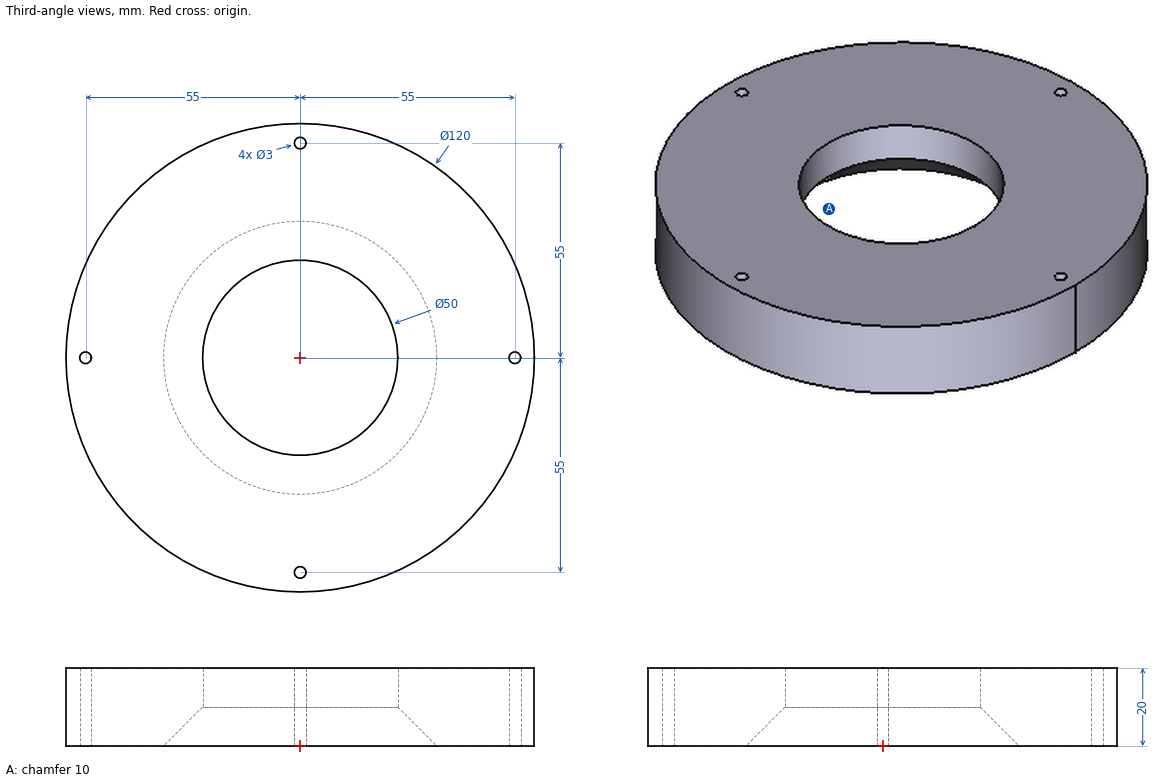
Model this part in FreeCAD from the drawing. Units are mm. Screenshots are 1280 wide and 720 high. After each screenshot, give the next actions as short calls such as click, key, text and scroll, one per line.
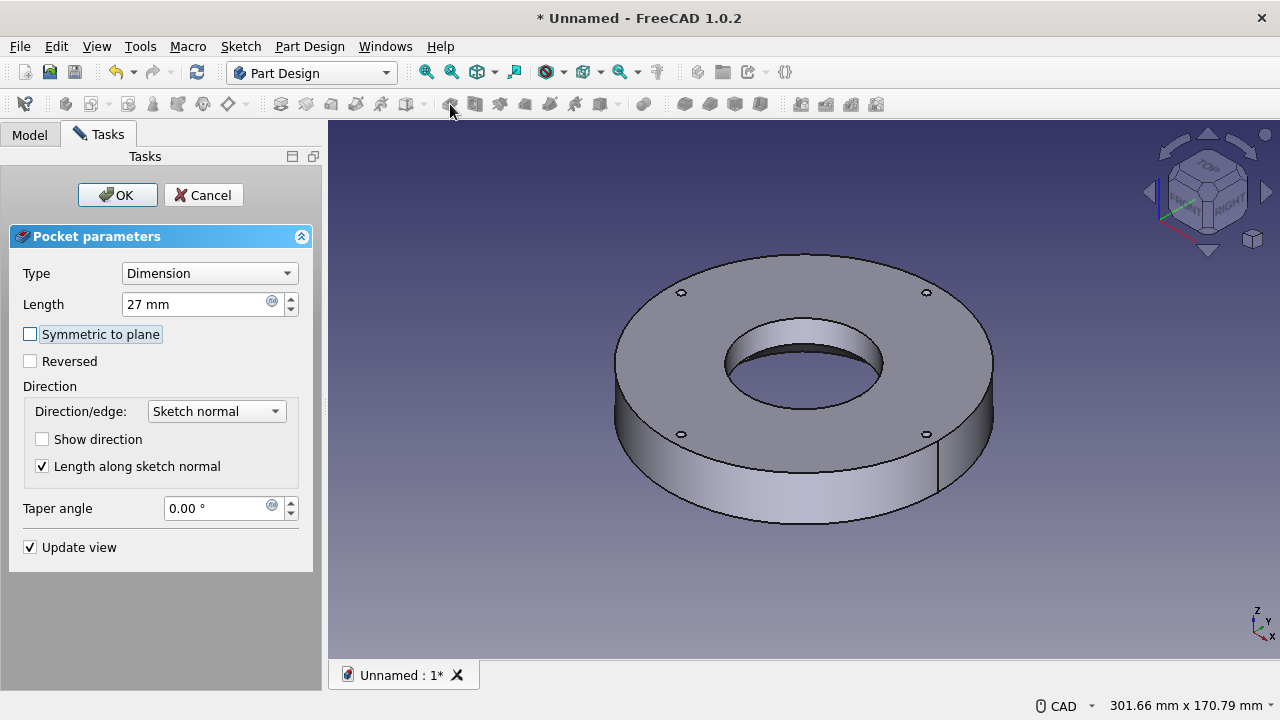
click(118, 195)